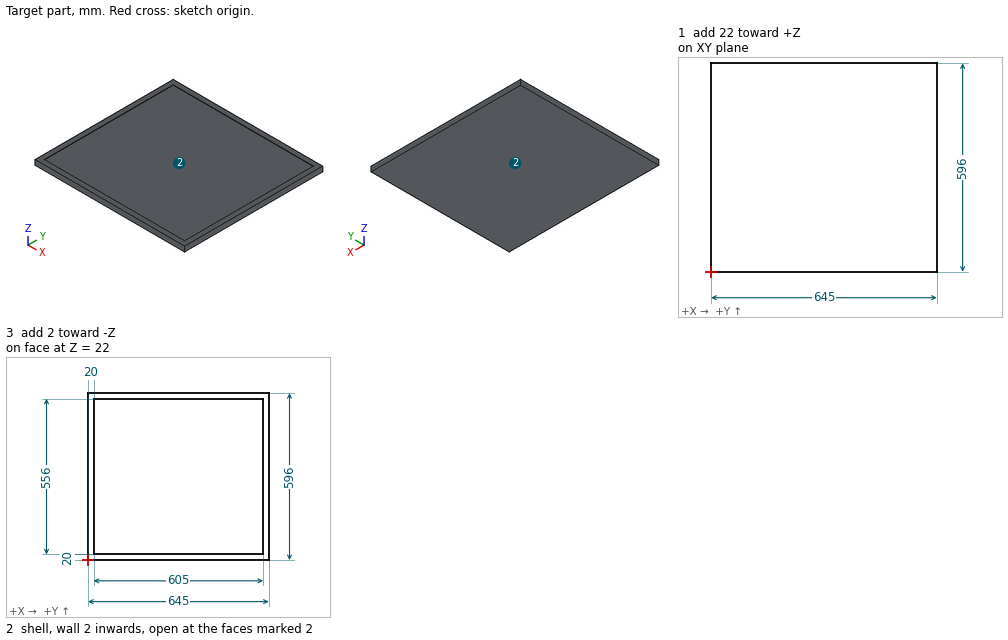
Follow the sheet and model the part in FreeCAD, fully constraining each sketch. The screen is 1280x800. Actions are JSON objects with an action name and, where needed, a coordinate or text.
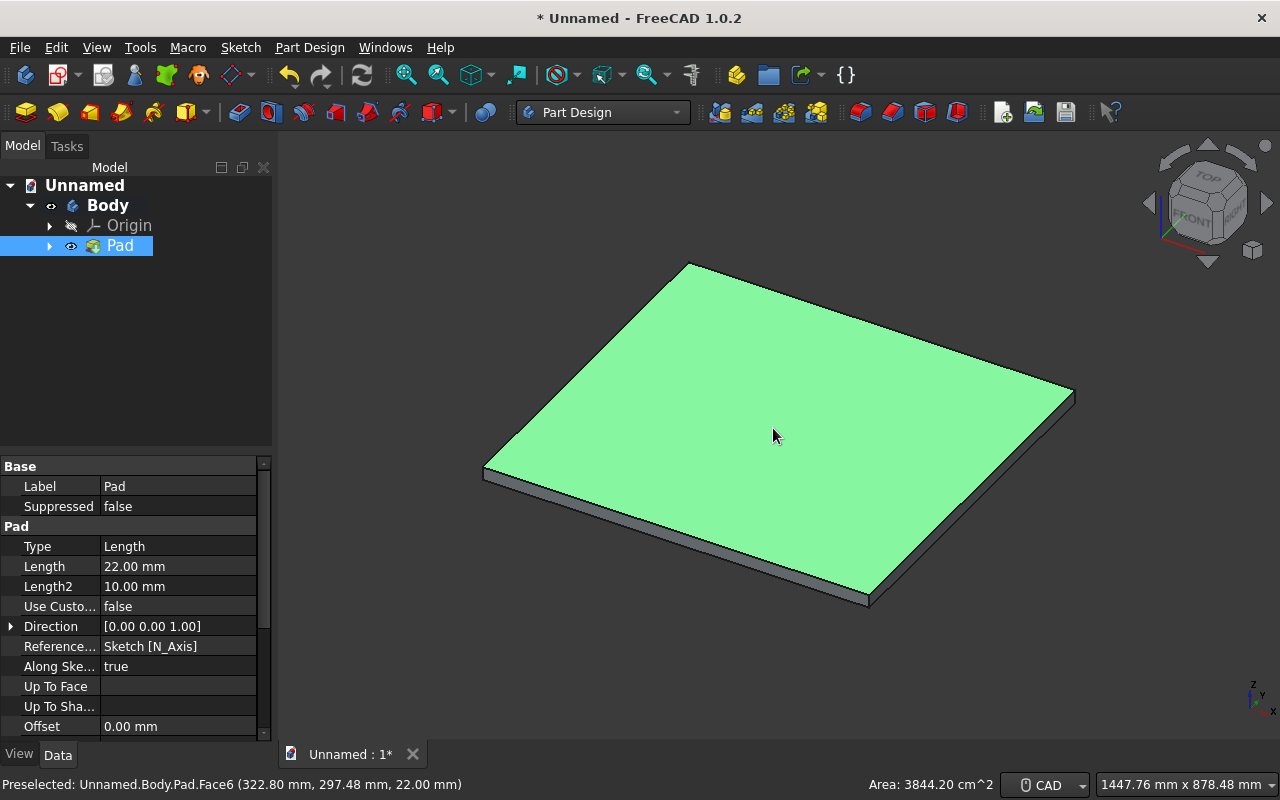
{"action": "left_click", "coordinate": [958, 112]}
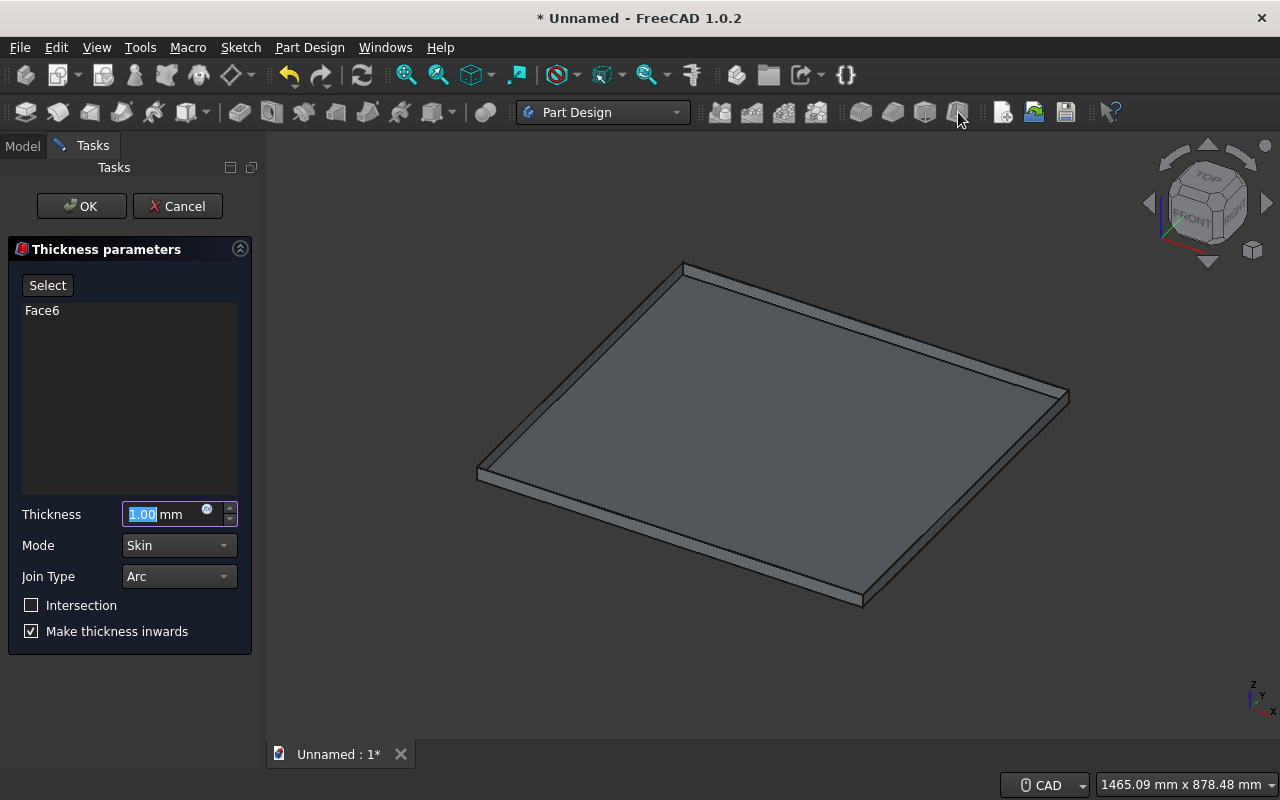
{"action": "type", "text": "2"}
{"action": "key", "text": "Tab"}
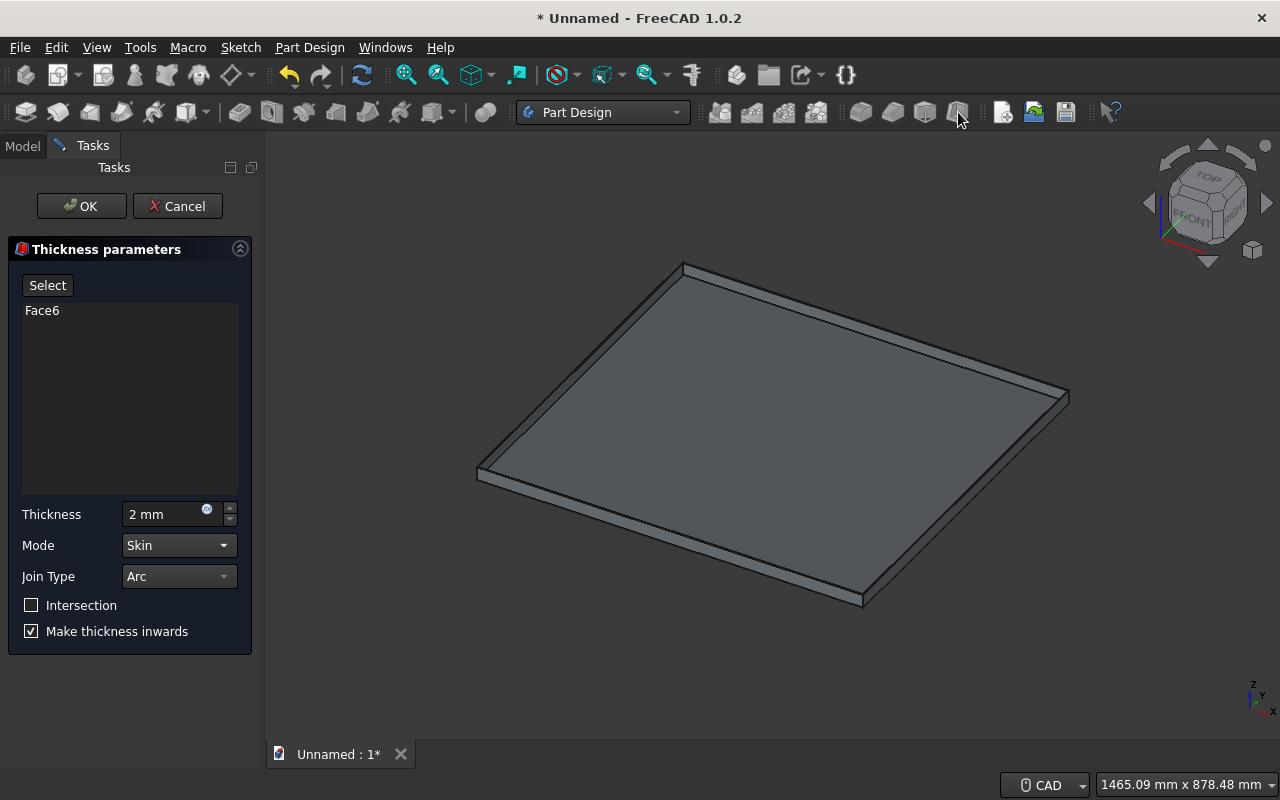
{"action": "left_click", "coordinate": [180, 576]}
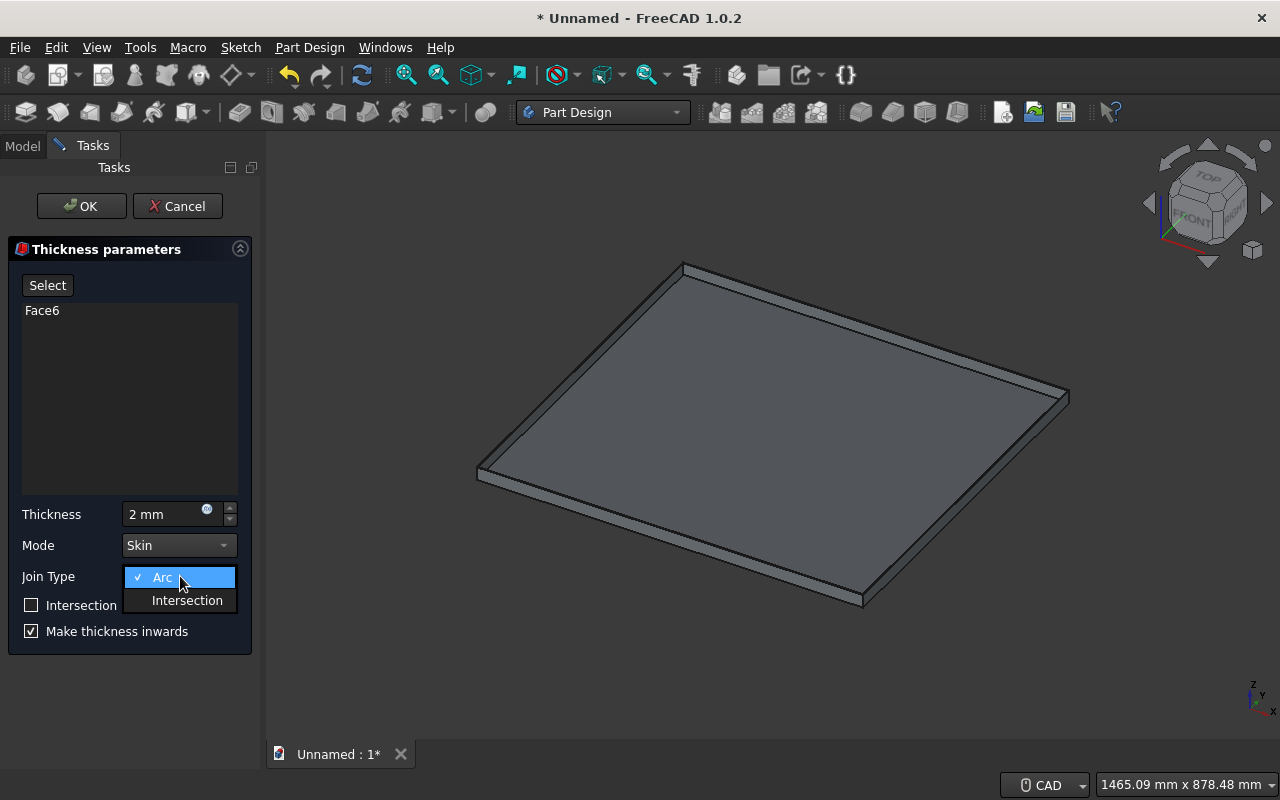
{"action": "left_click", "coordinate": [179, 600]}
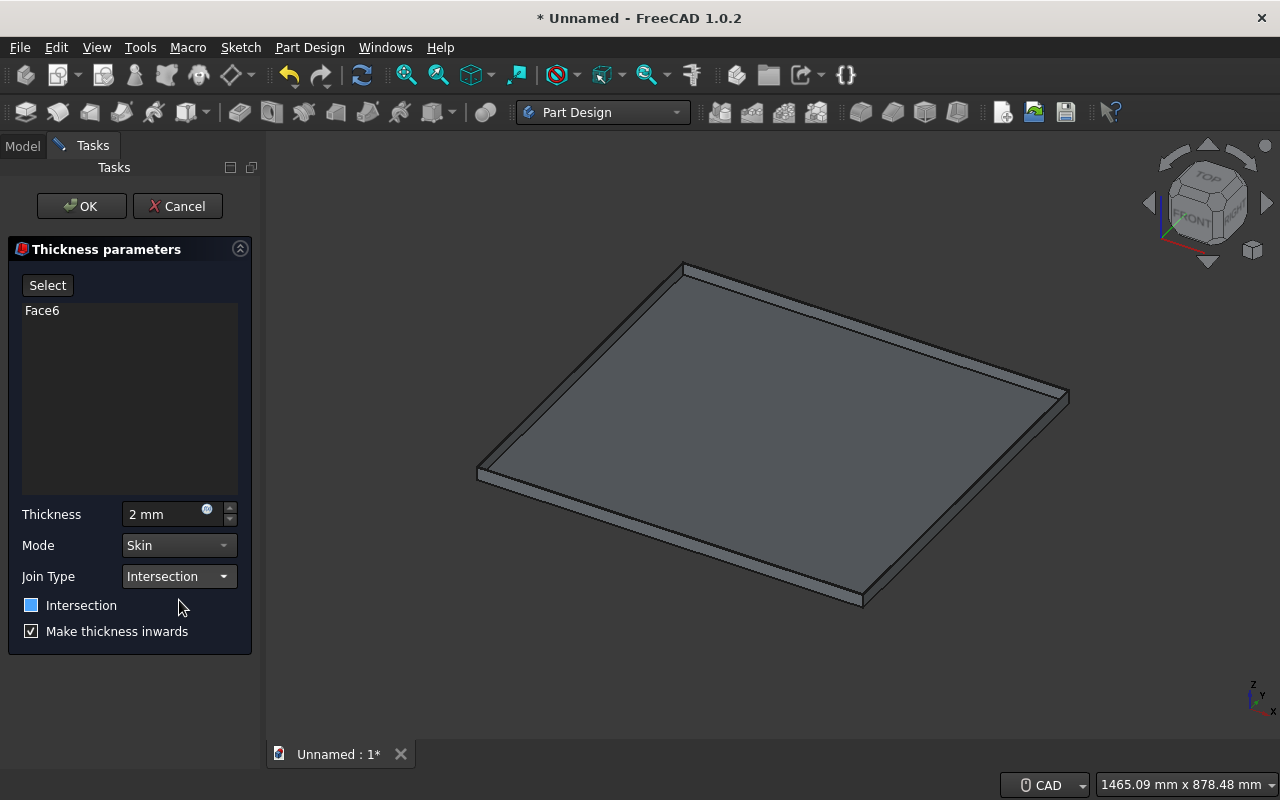
{"action": "left_click", "coordinate": [82, 206]}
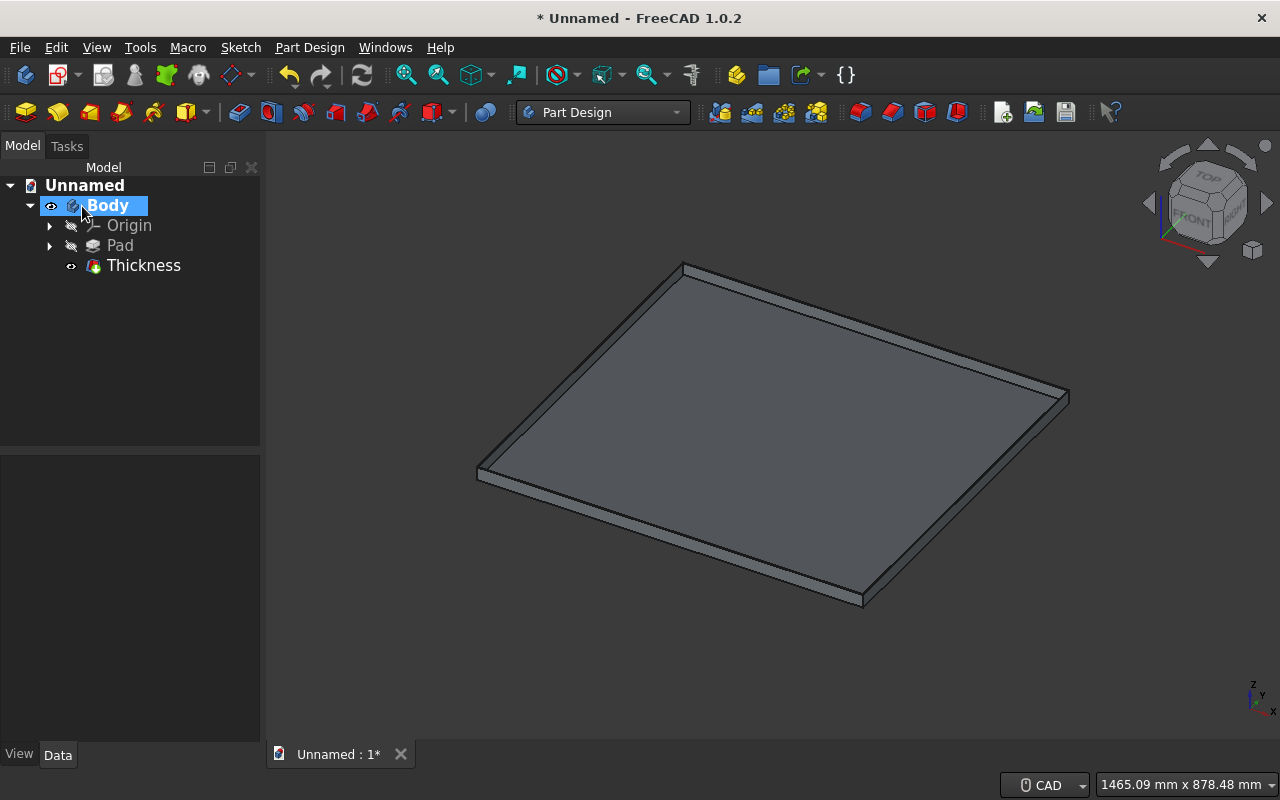
{"action": "scroll", "coordinate": [606, 508], "scroll_direction": "up", "scroll_amount": 15}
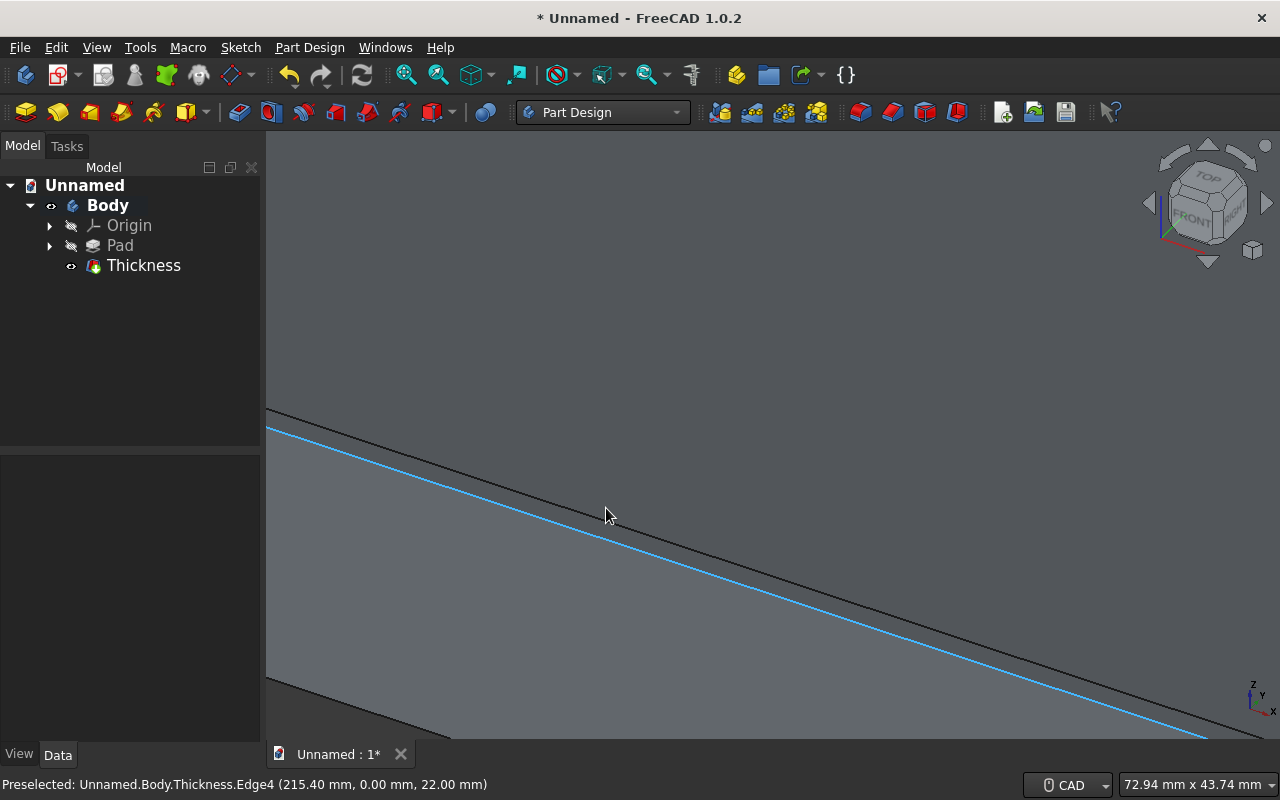
{"action": "left_click", "coordinate": [598, 524]}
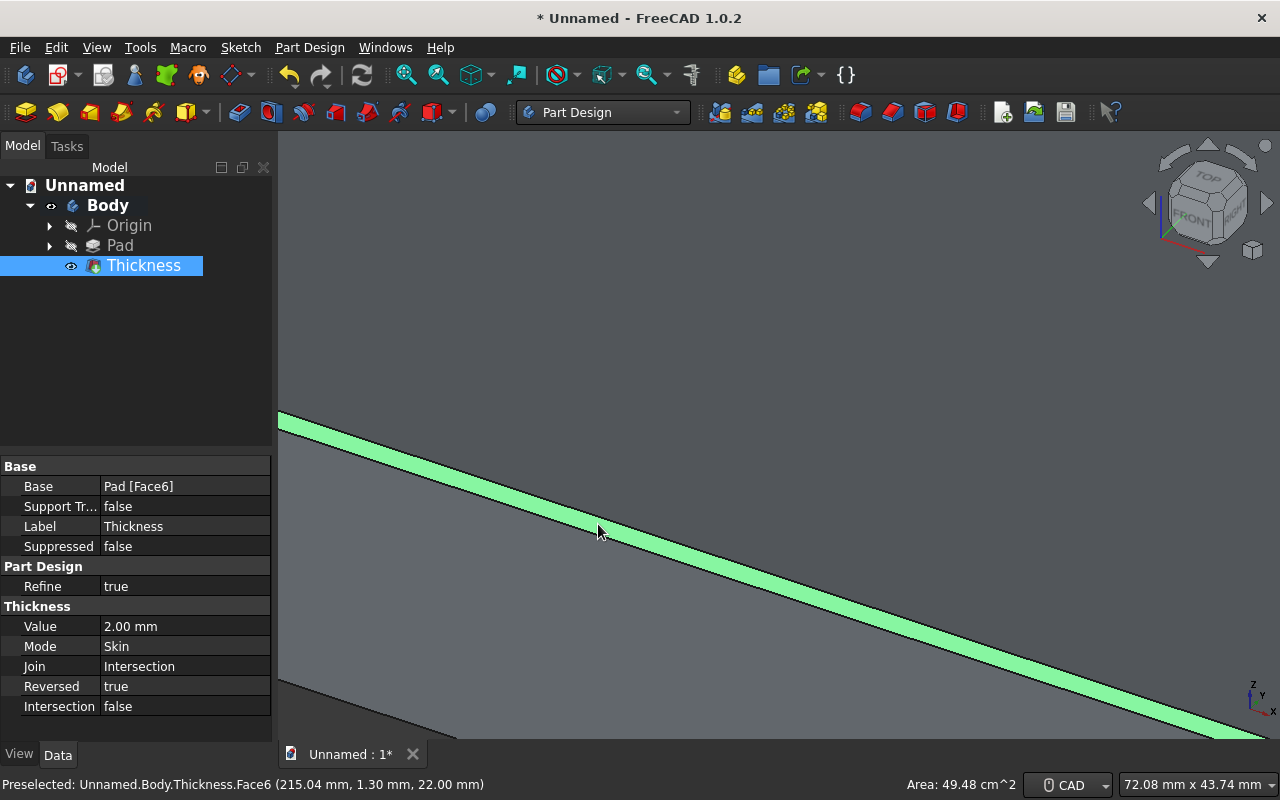
{"action": "left_click", "coordinate": [58, 76]}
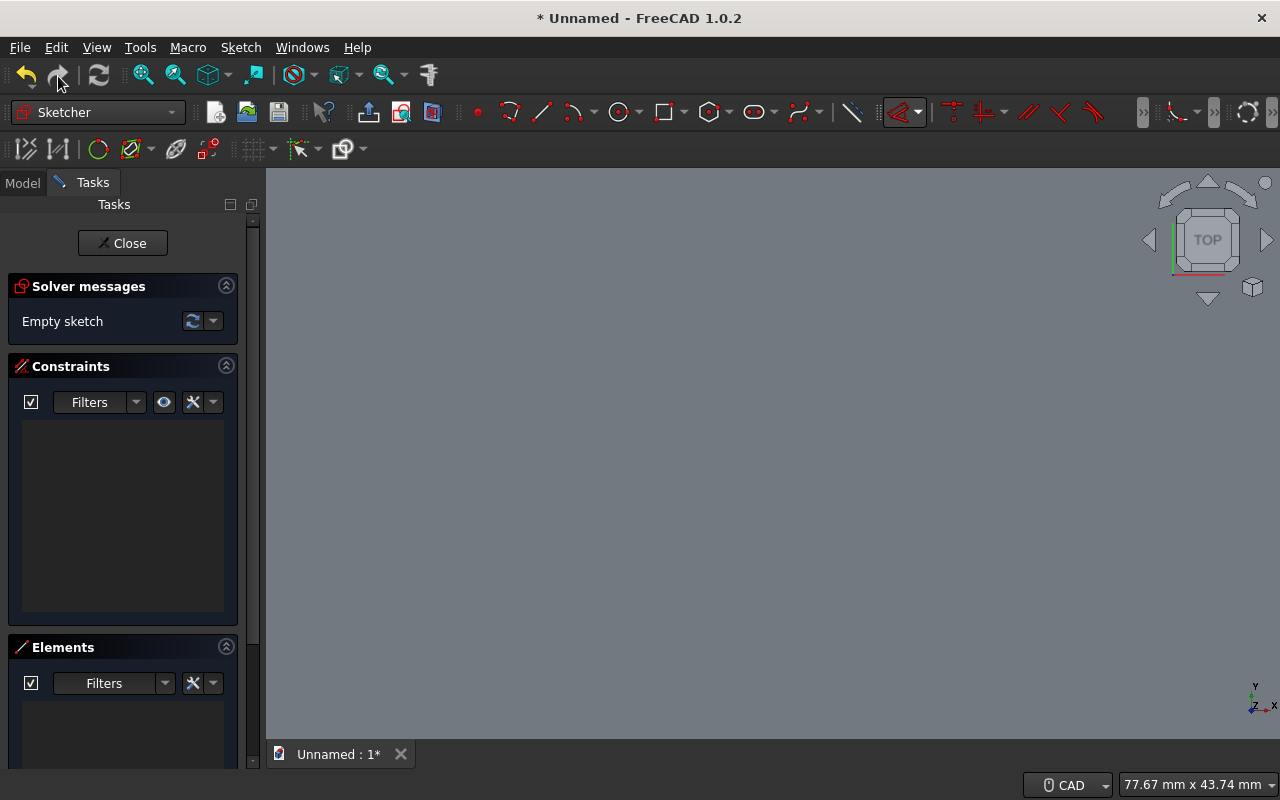
{"action": "scroll", "coordinate": [585, 566], "scroll_direction": "down", "scroll_amount": 15}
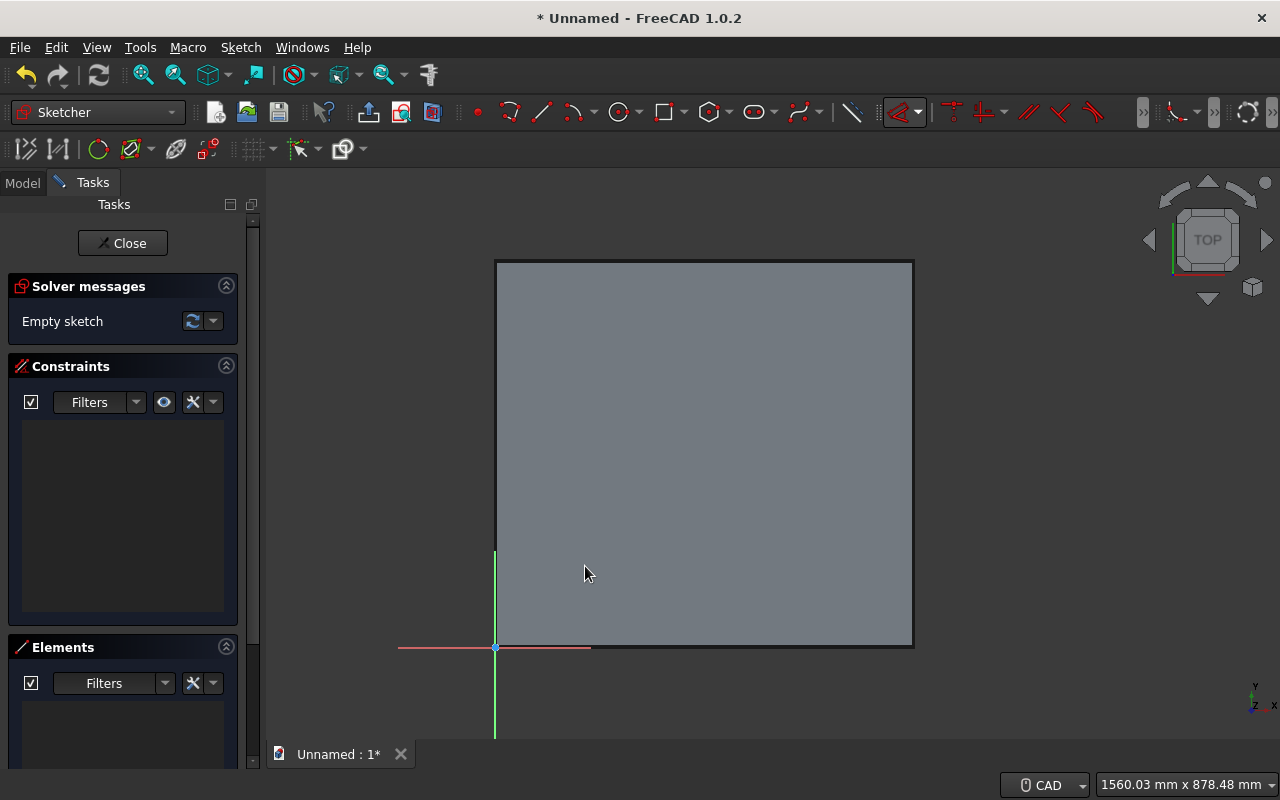
{"action": "left_click", "coordinate": [664, 112]}